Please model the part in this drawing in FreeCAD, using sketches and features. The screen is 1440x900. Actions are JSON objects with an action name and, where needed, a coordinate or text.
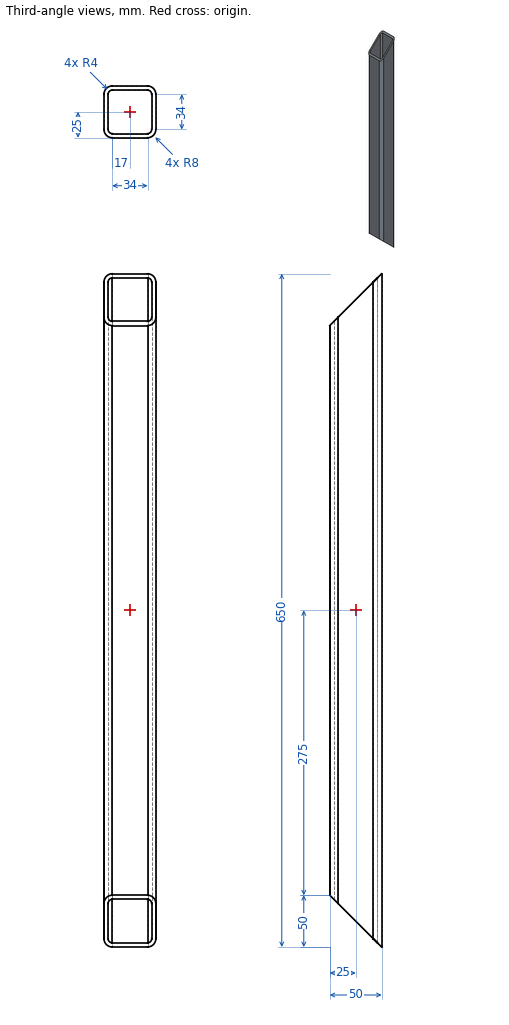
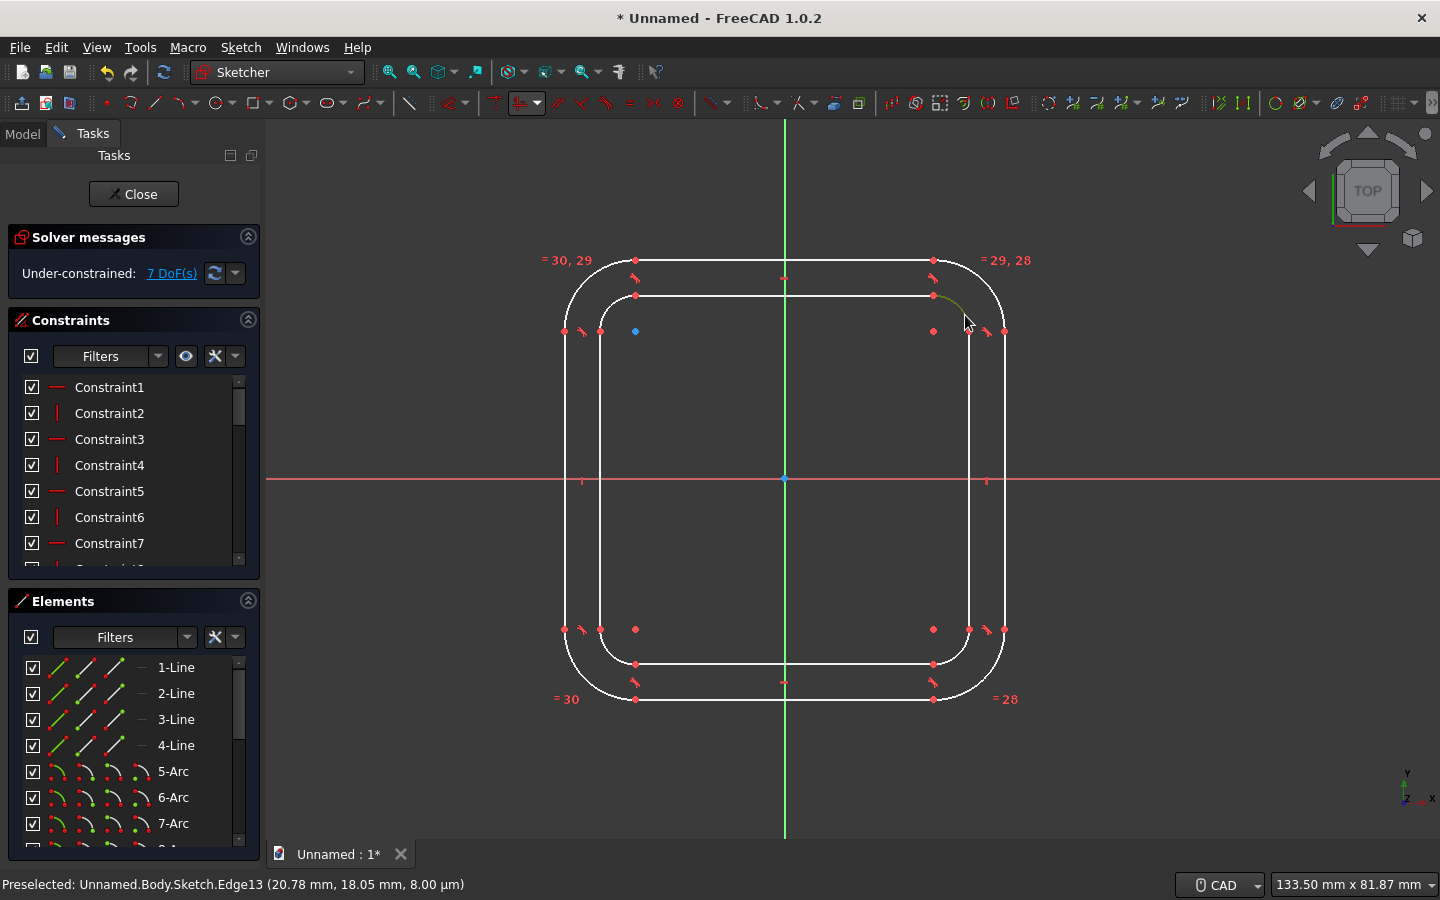
{"action": "left_click", "coordinate": [619, 300]}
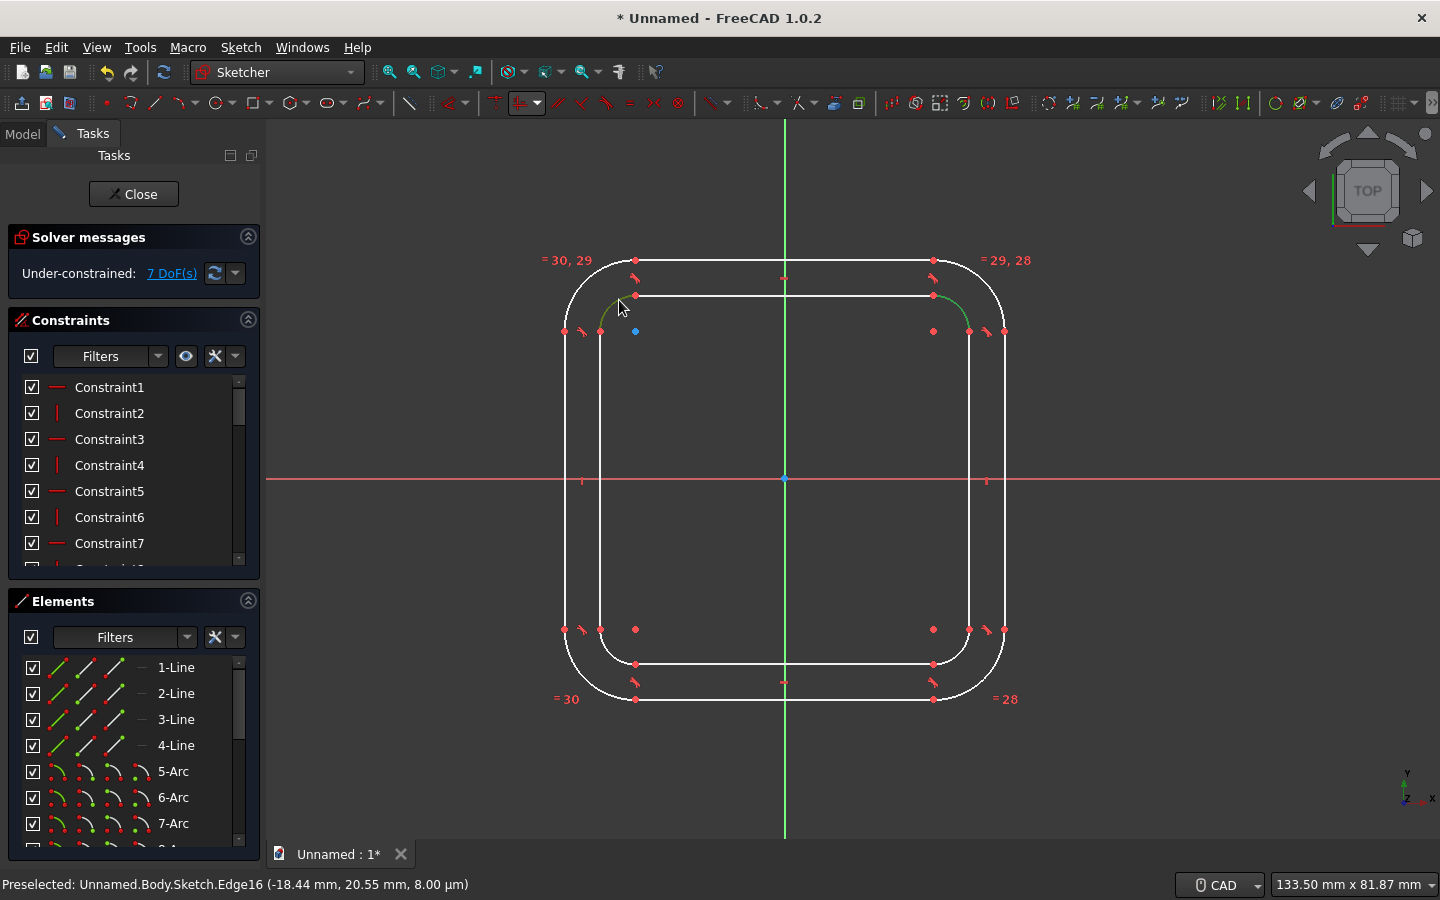
{"action": "left_click", "coordinate": [630, 104]}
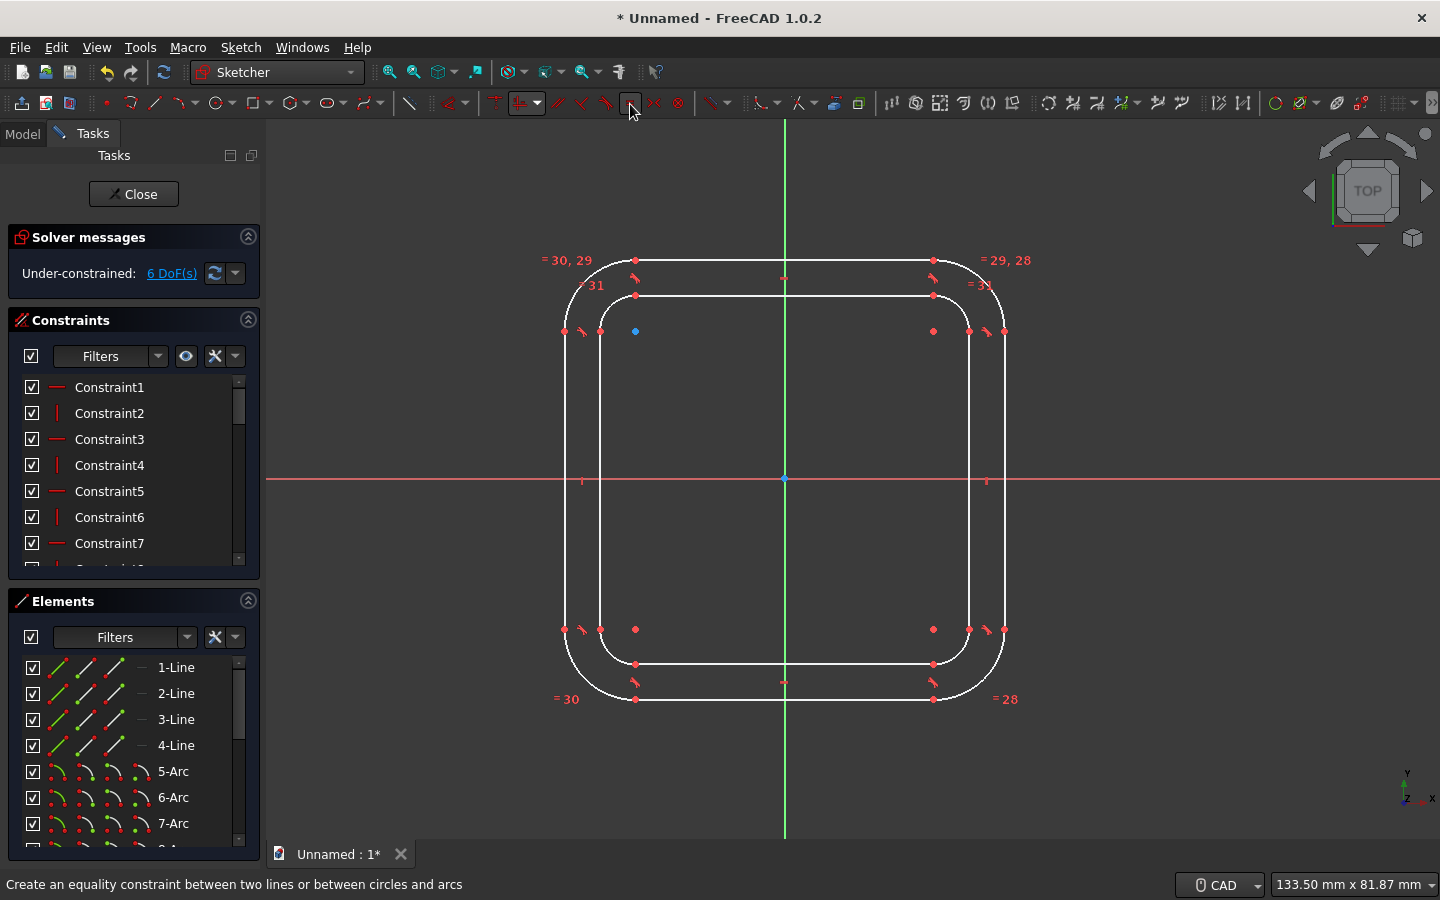
{"action": "left_click", "coordinate": [966, 692]}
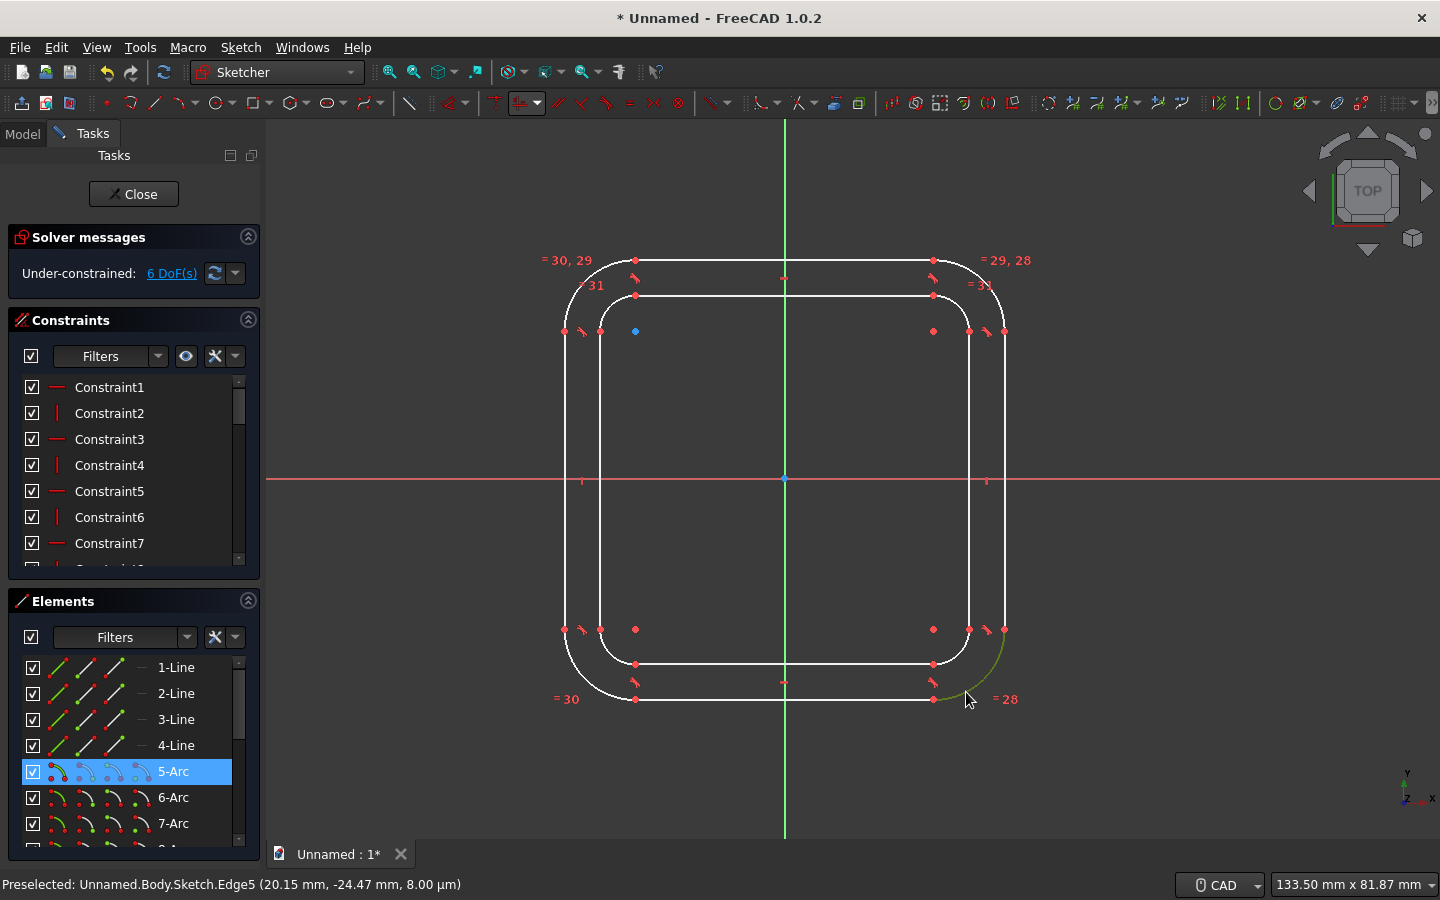
{"action": "key", "text": "k r"}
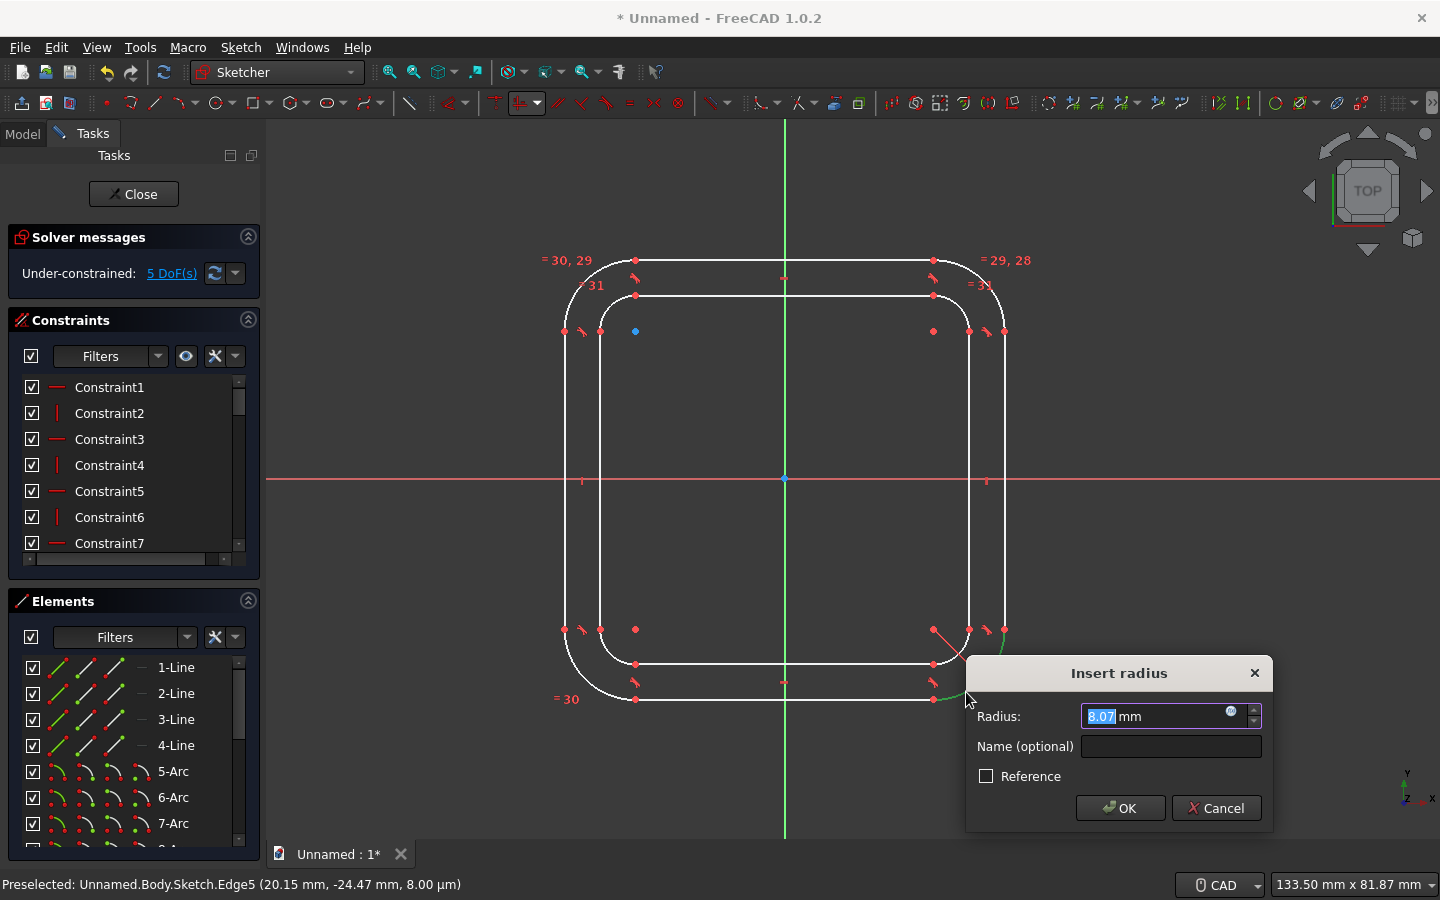
{"action": "type", "text": "8"}
{"action": "key", "text": "Return"}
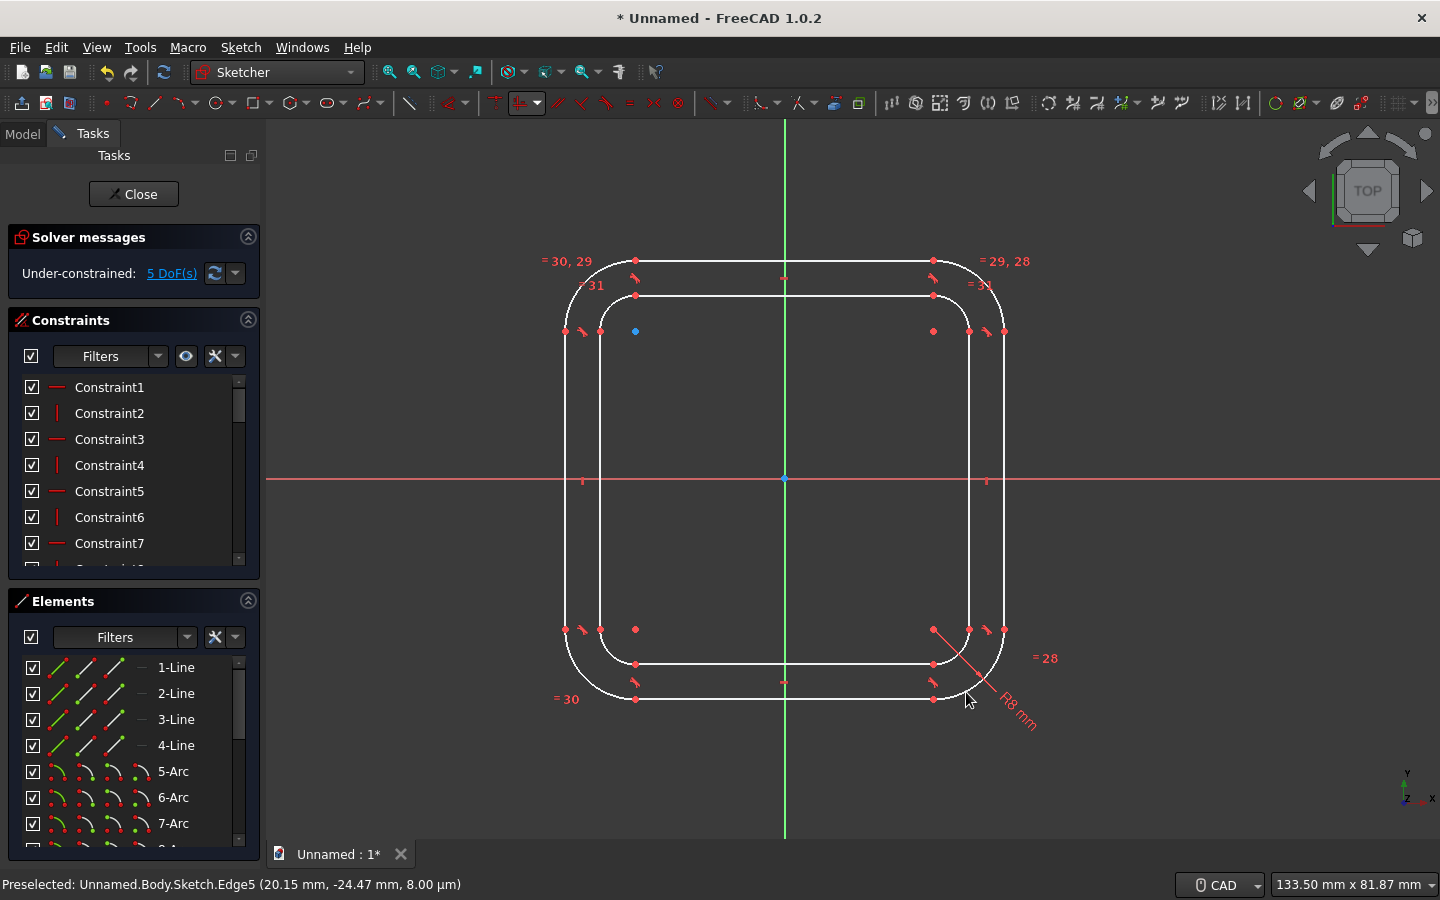
{"action": "left_click", "coordinate": [965, 315]}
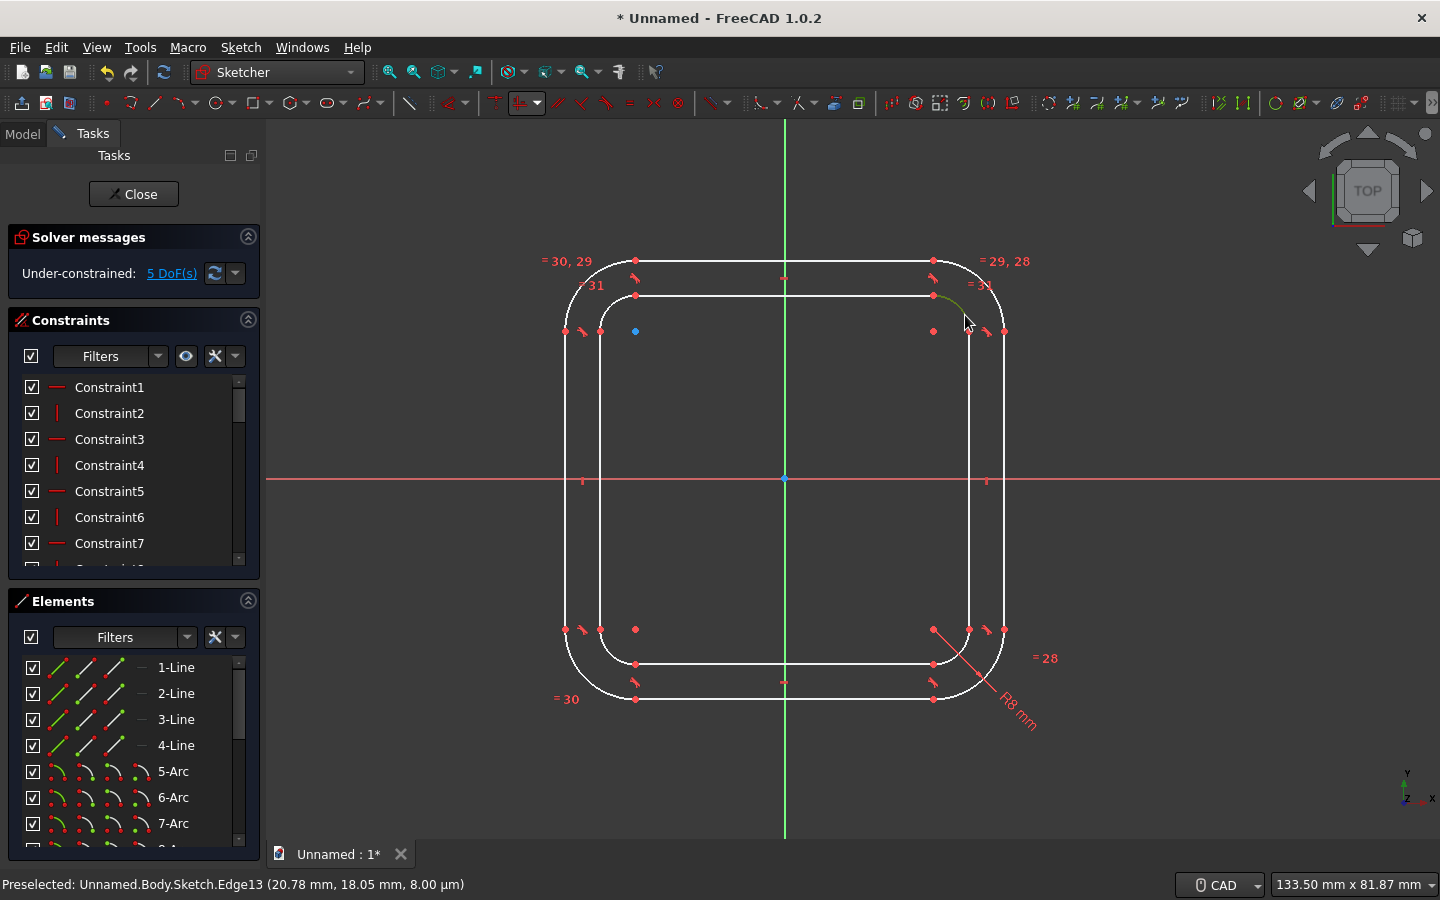
{"action": "key", "text": "k r"}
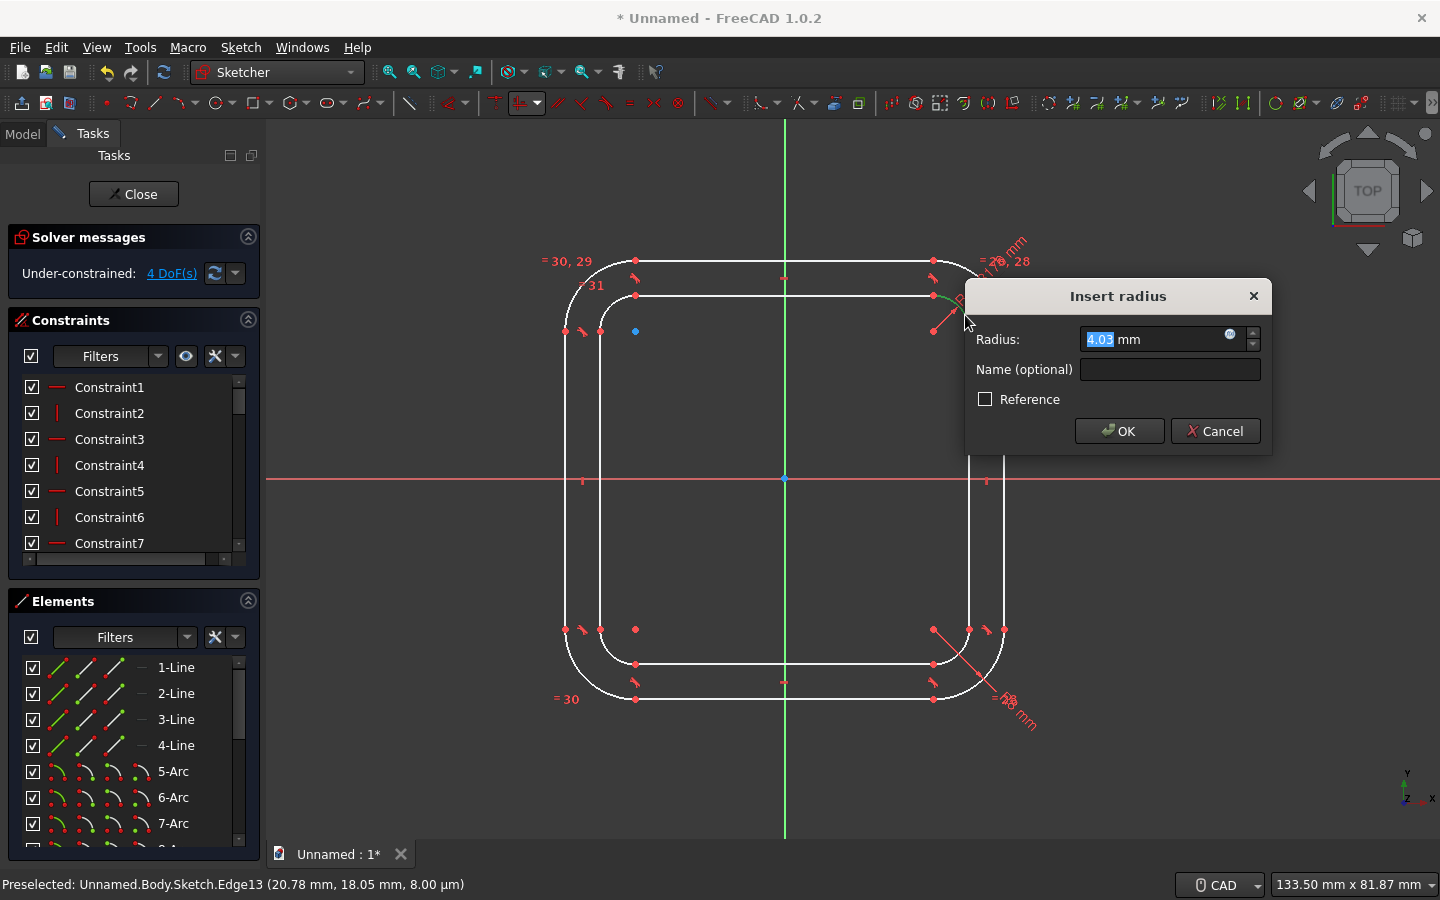
{"action": "type", "text": "4"}
{"action": "key", "text": "Return"}